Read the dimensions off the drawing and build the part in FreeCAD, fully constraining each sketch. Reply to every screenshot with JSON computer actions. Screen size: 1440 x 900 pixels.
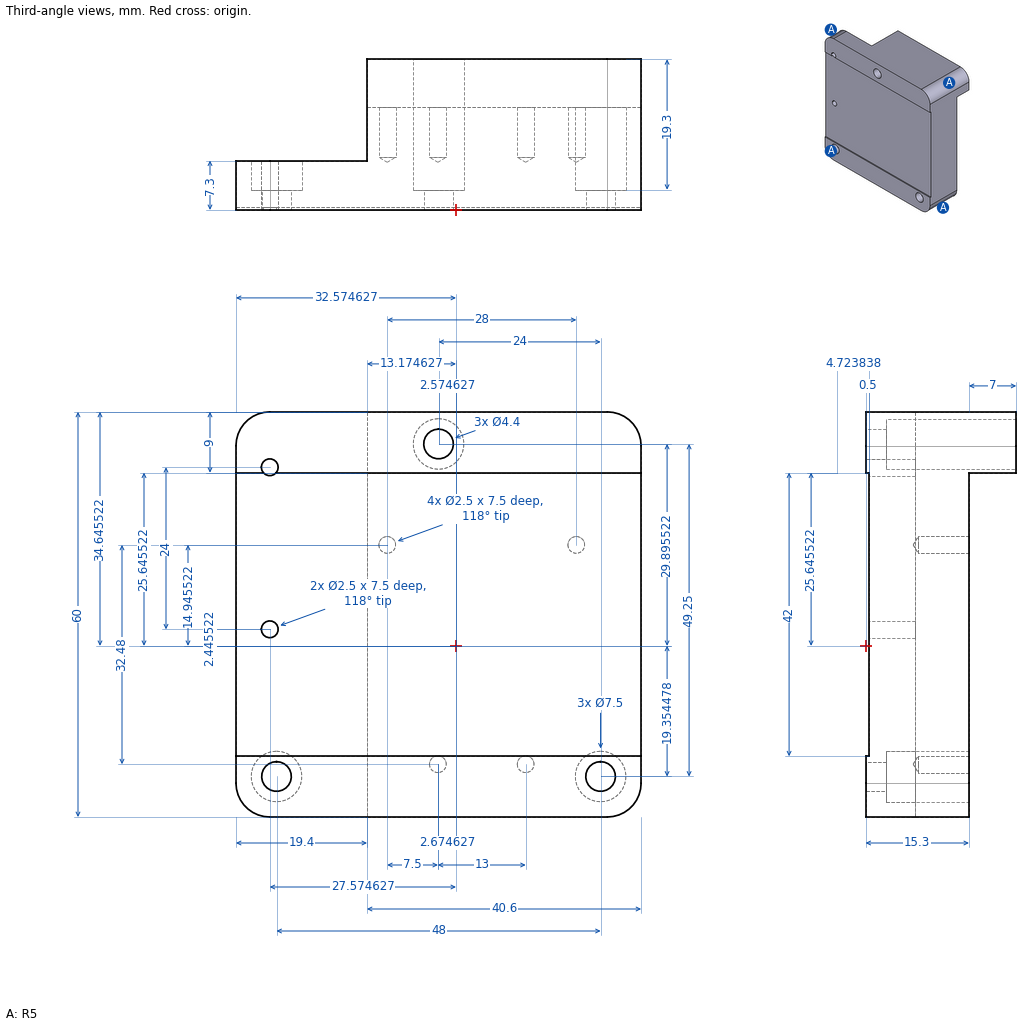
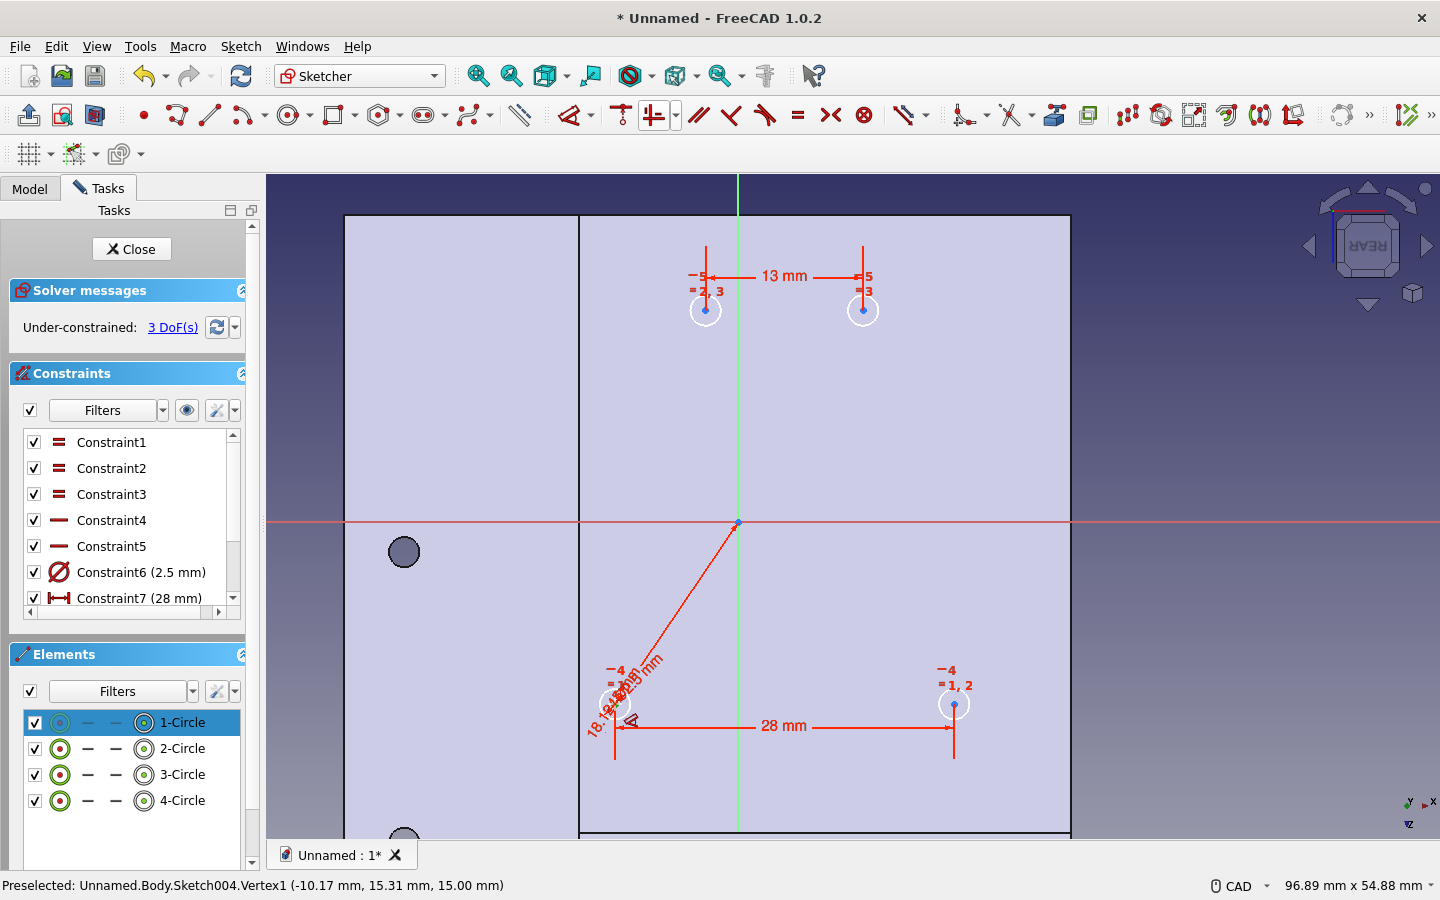
{"action": "left_click", "coordinate": [706, 311]}
{"action": "left_click", "coordinate": [660, 738]}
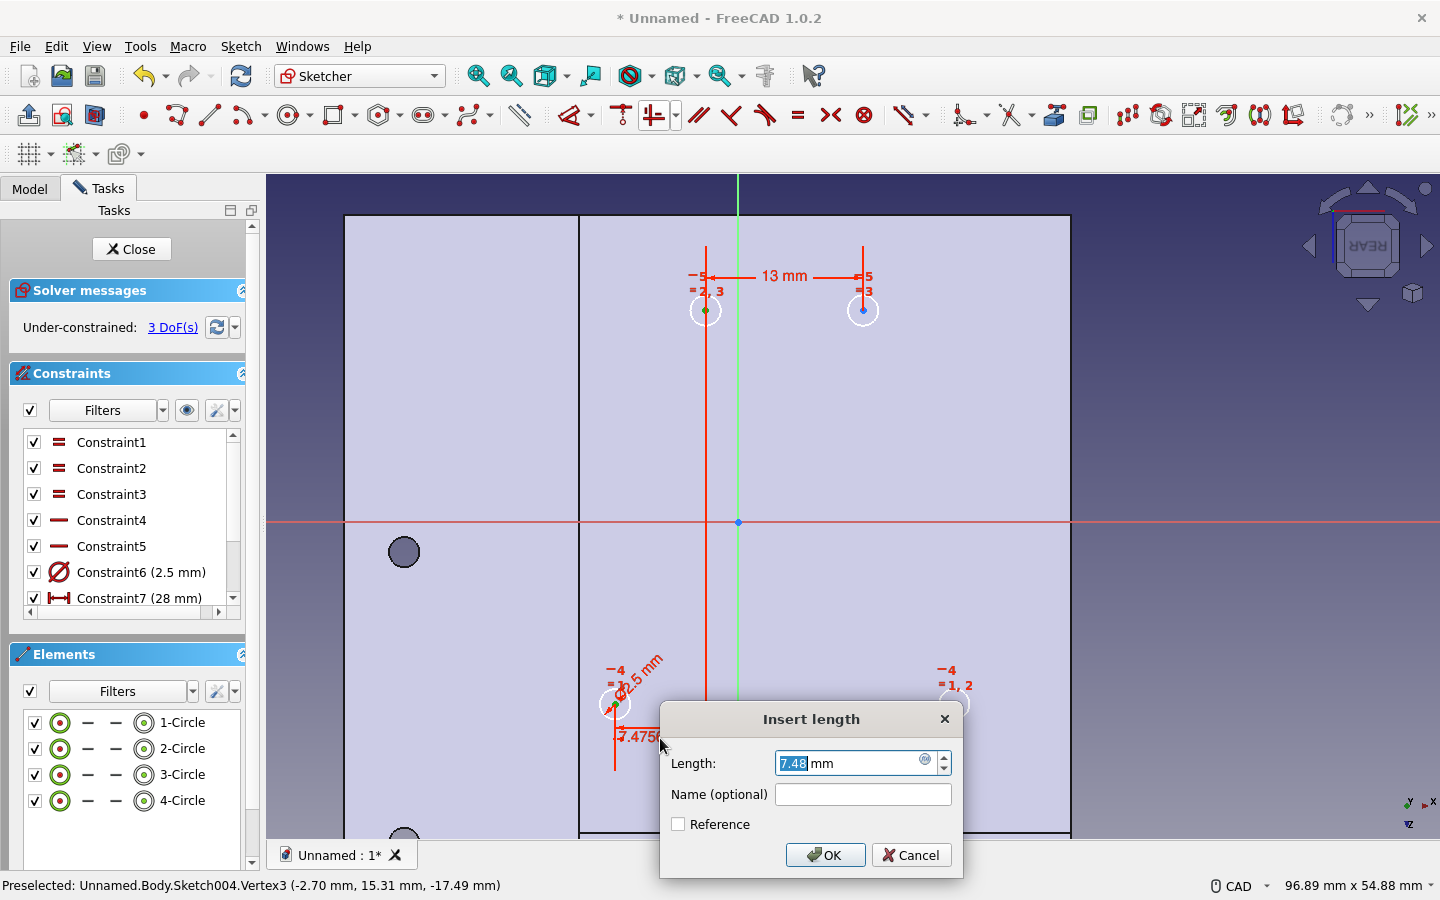
{"action": "type", "text": "7.5"}
{"action": "key", "text": "Return"}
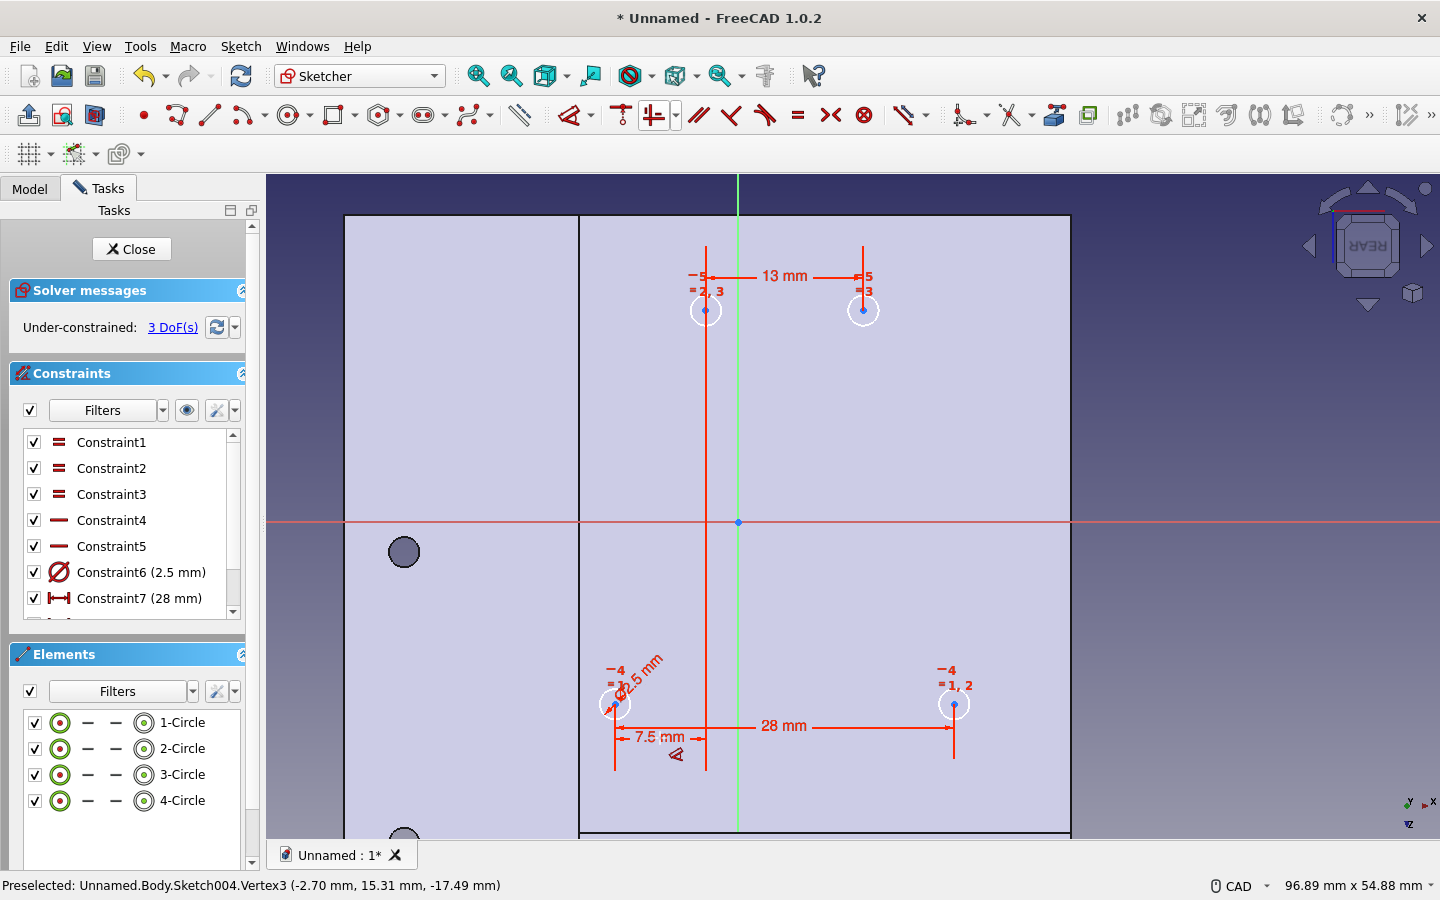
{"action": "left_click", "coordinate": [615, 704]}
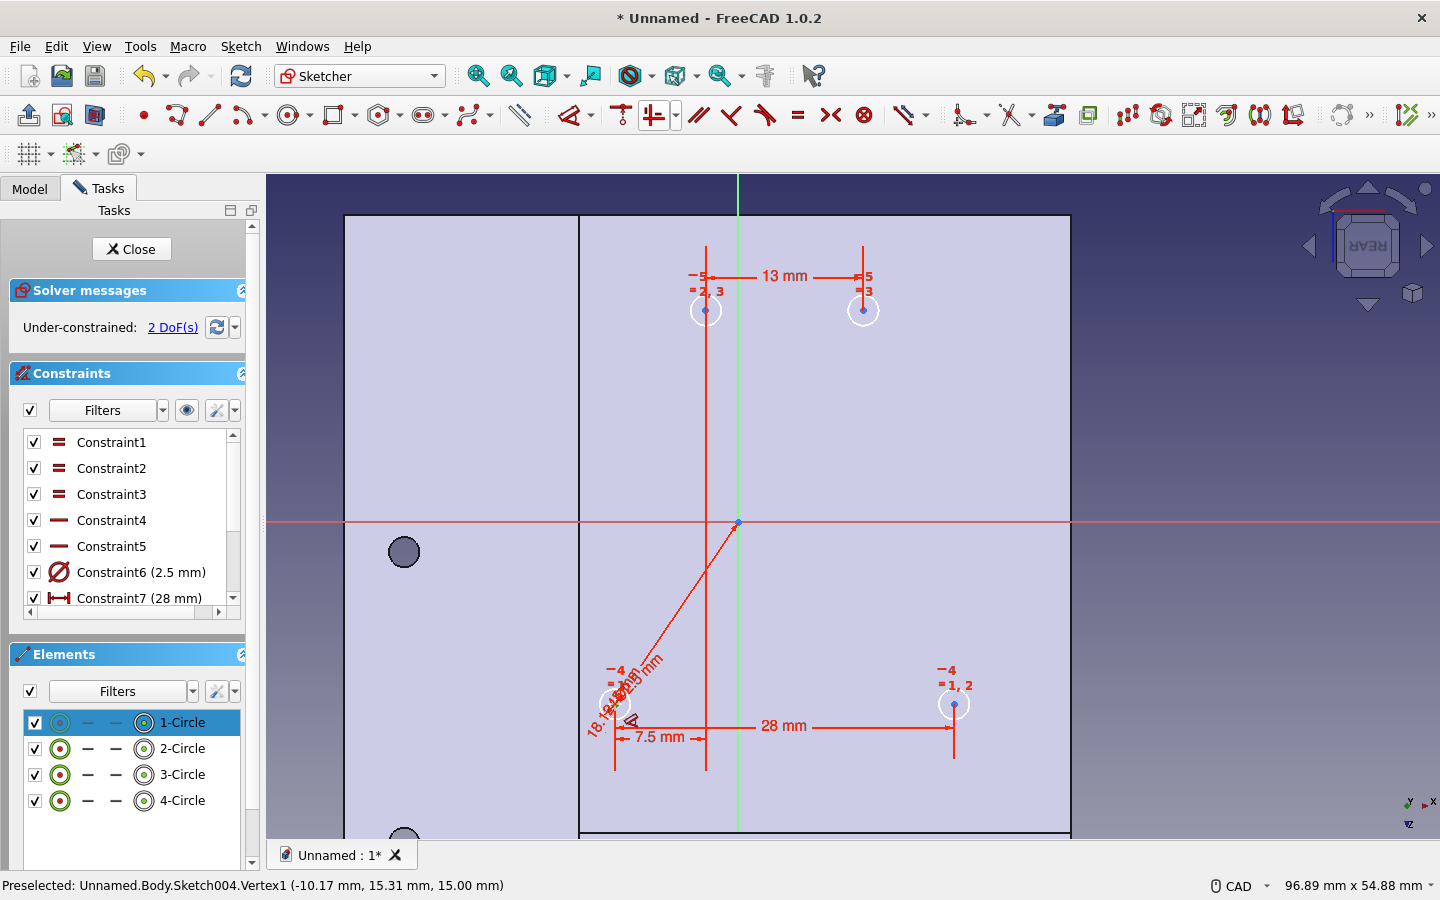
{"action": "left_click", "coordinate": [706, 311]}
{"action": "left_click", "coordinate": [581, 507]}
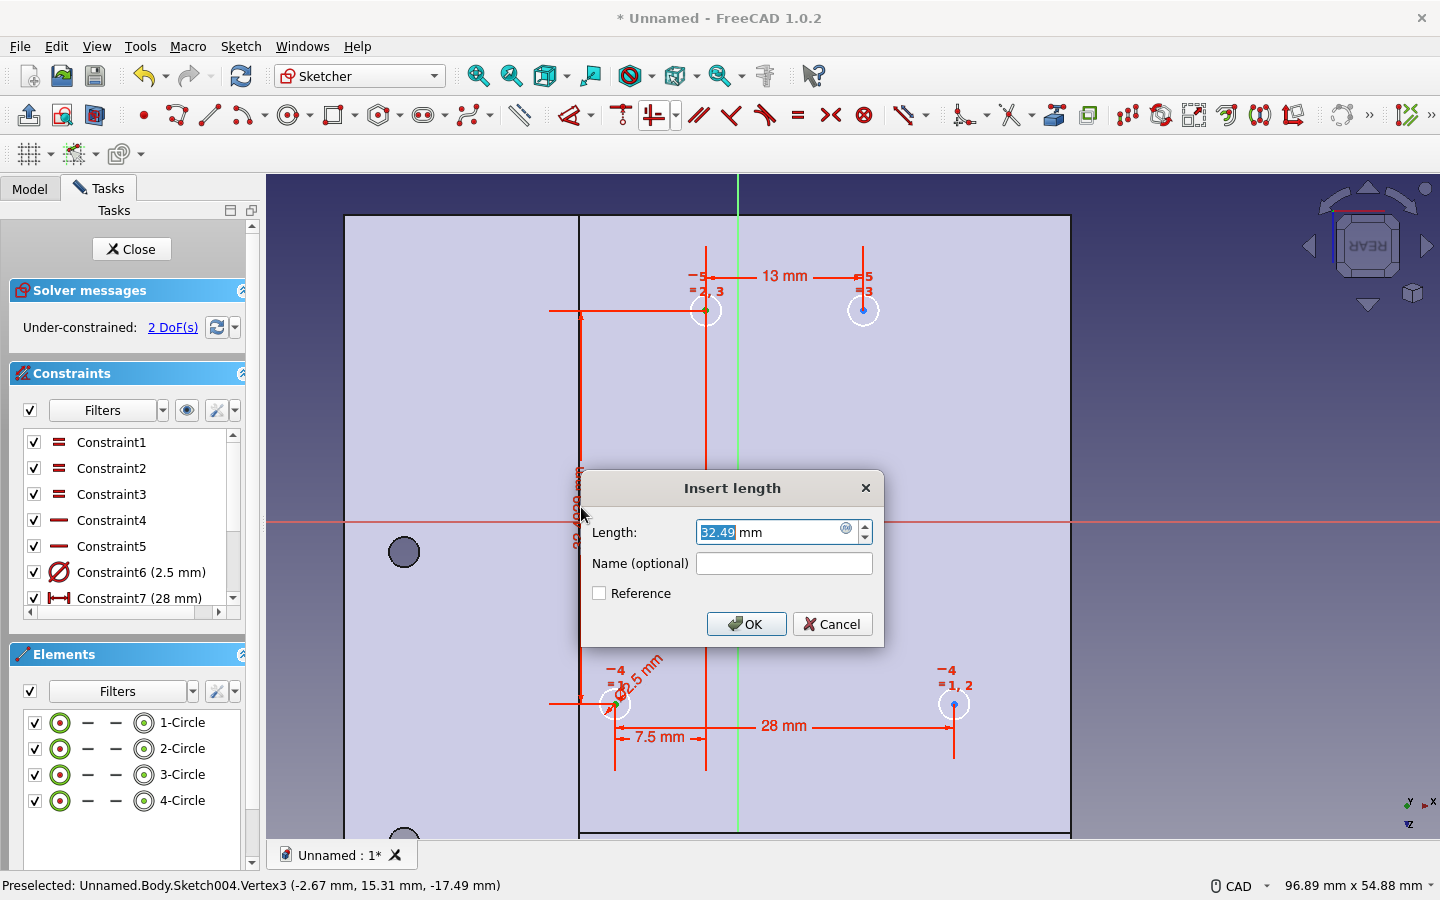
{"action": "type", "text": "32.48"}
{"action": "key", "text": "Return"}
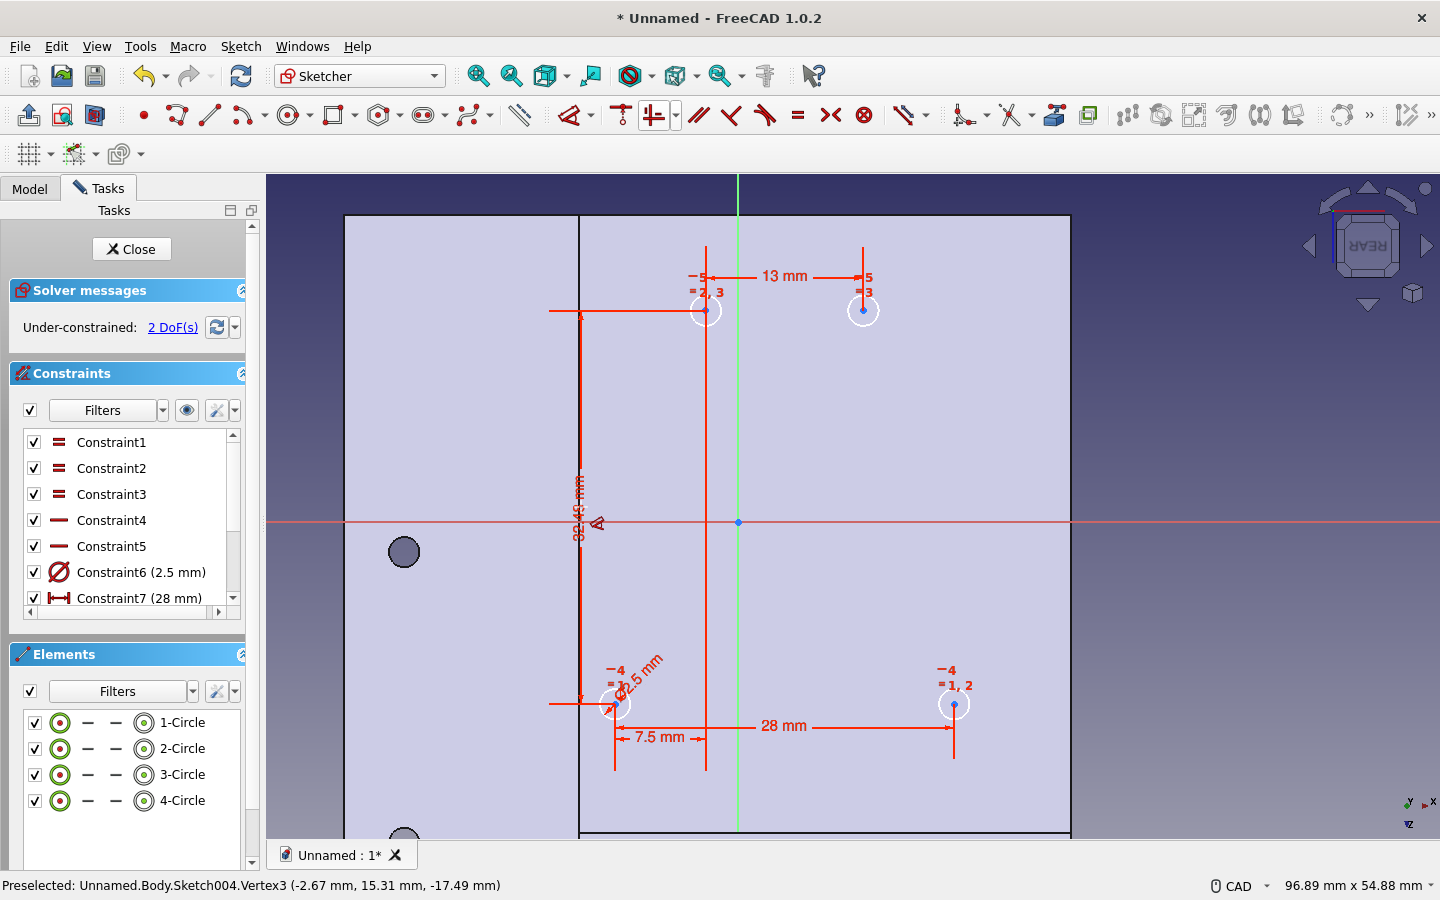
{"action": "scroll", "coordinate": [706, 311], "scroll_direction": "up", "scroll_amount": 2}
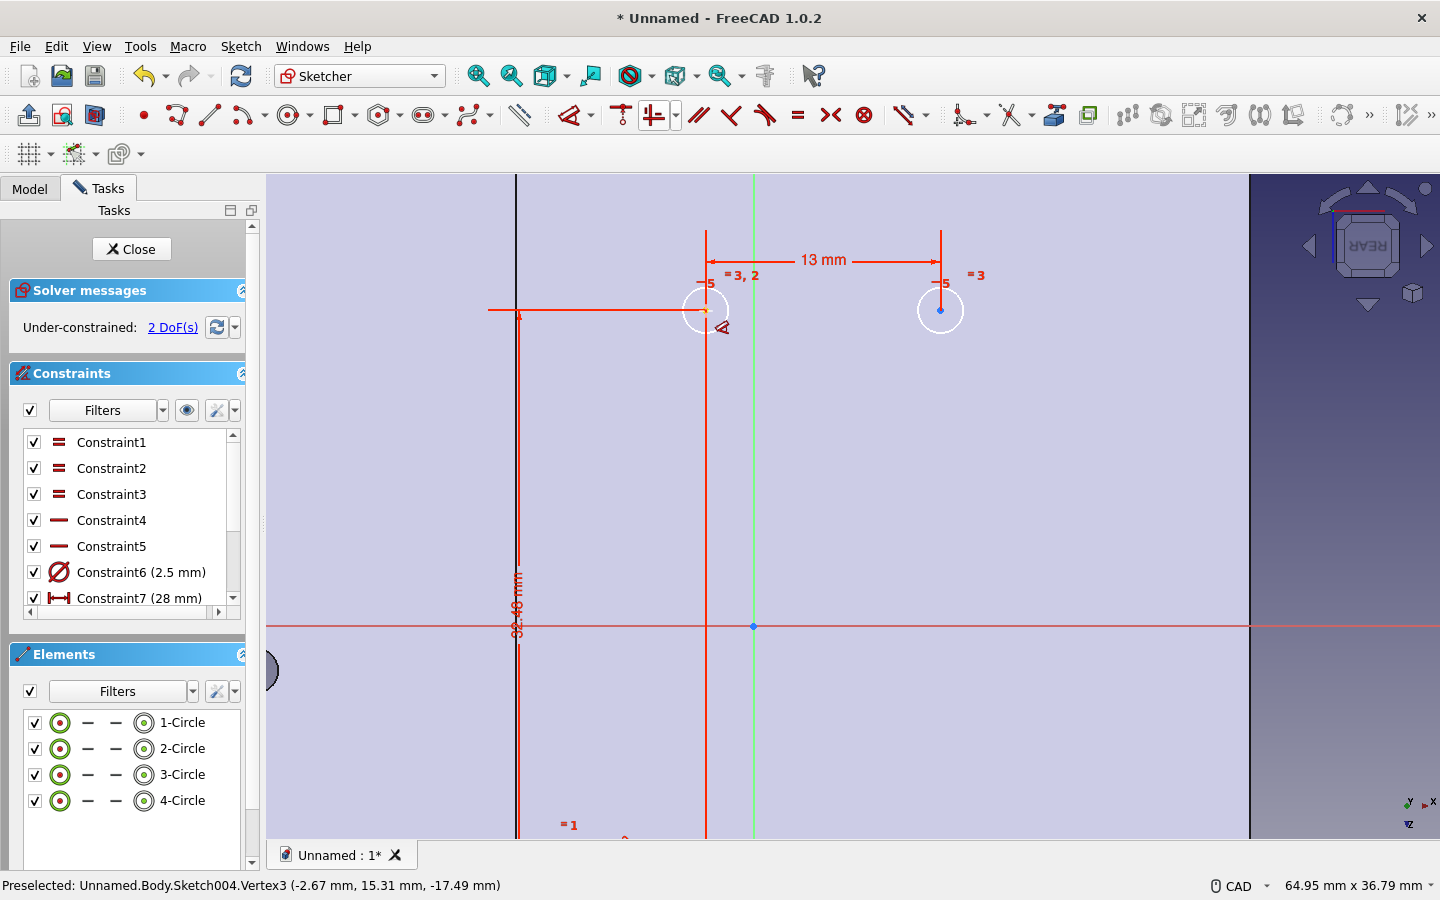
{"action": "left_click", "coordinate": [706, 310]}
{"action": "left_click", "coordinate": [730, 276]}